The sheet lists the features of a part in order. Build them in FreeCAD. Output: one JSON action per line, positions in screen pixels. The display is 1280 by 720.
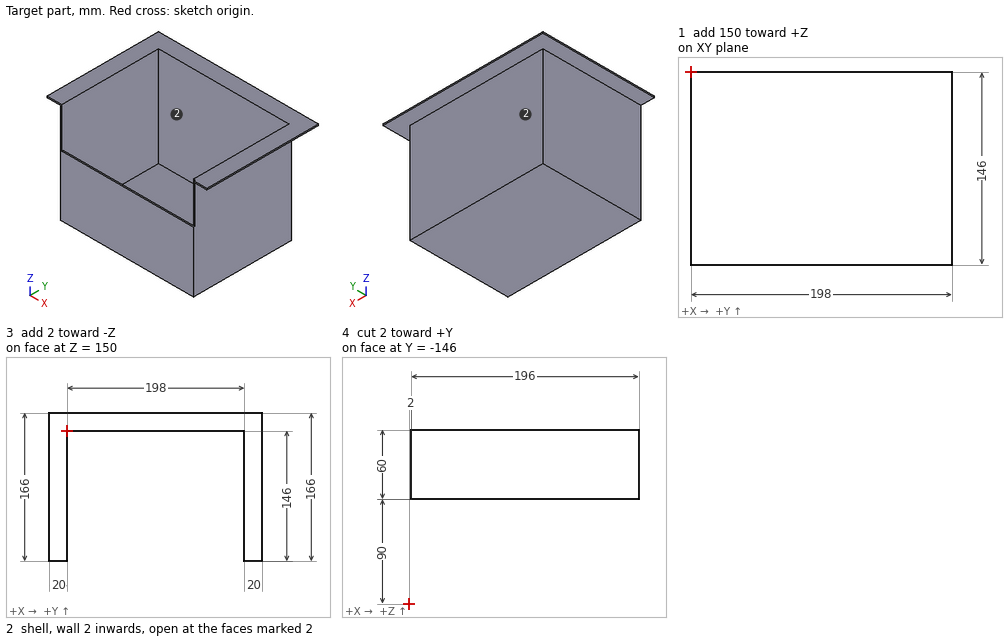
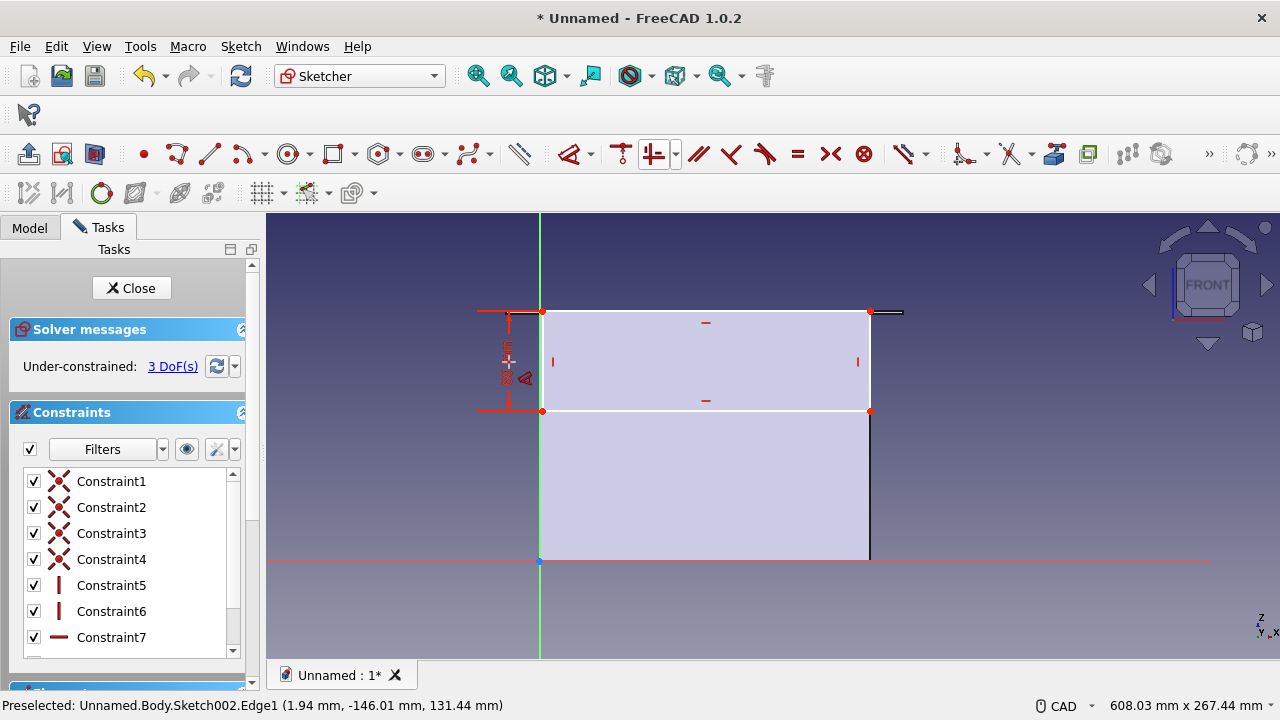
{"action": "scroll", "coordinate": [543, 311], "scroll_direction": "up", "scroll_amount": 13}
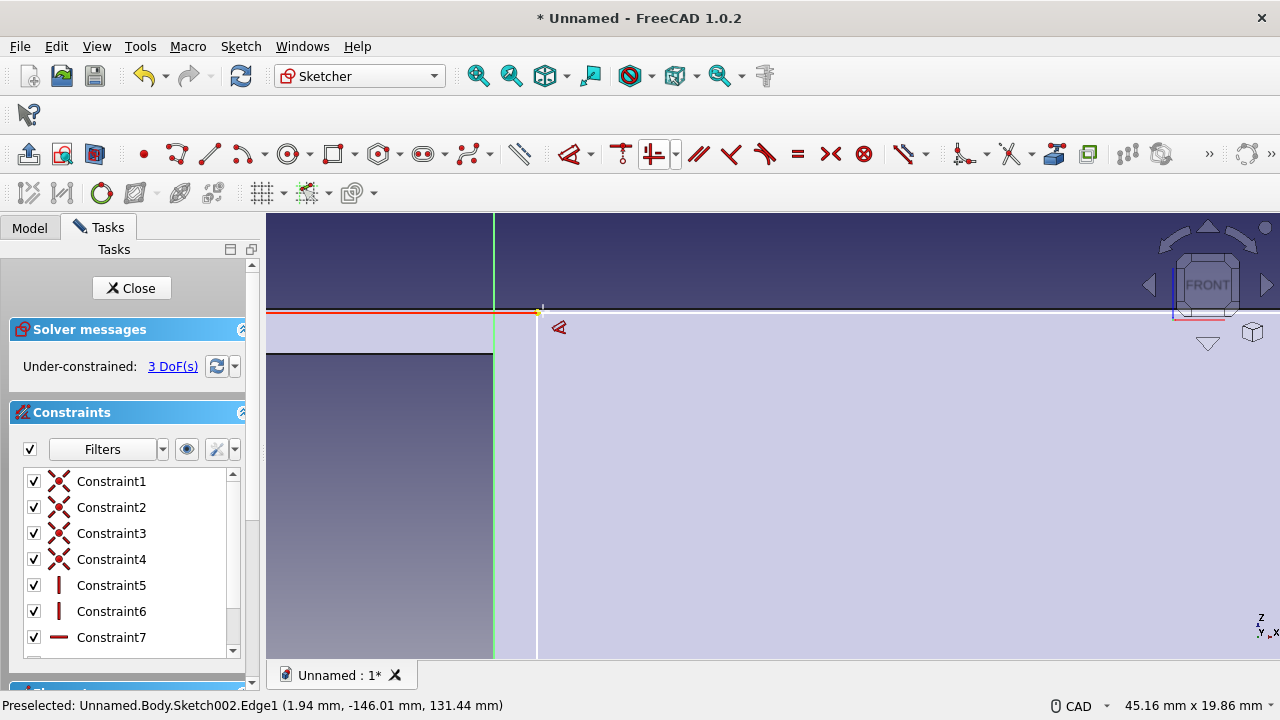
{"action": "left_click", "coordinate": [537, 313]}
{"action": "left_click", "coordinate": [515, 279]}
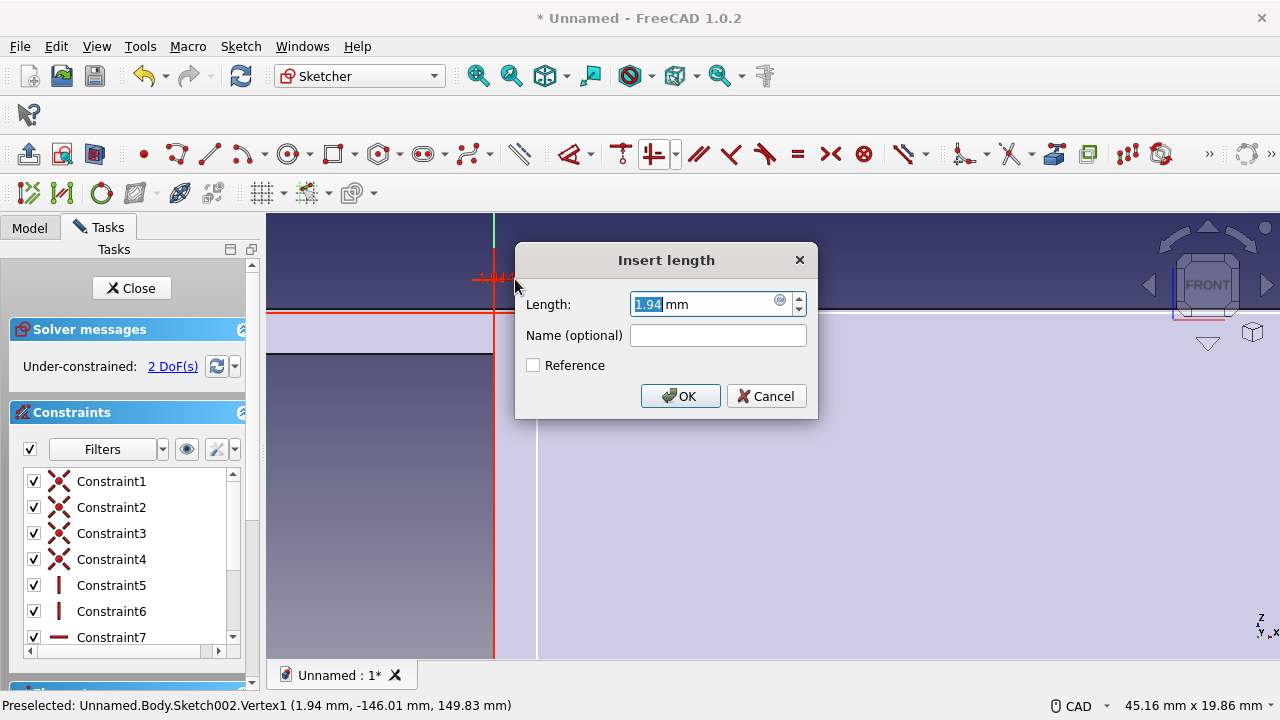
{"action": "type", "text": "2"}
{"action": "key", "text": "Return"}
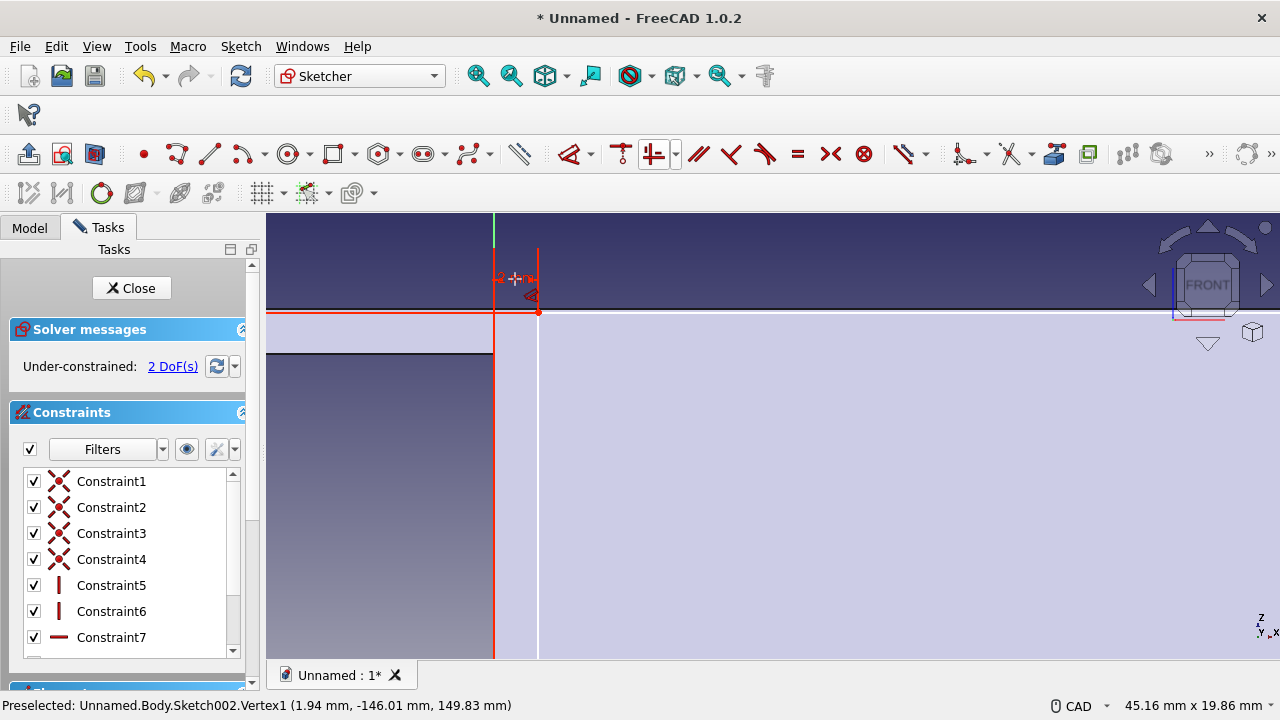
{"action": "scroll", "coordinate": [543, 311], "scroll_direction": "down", "scroll_amount": 13}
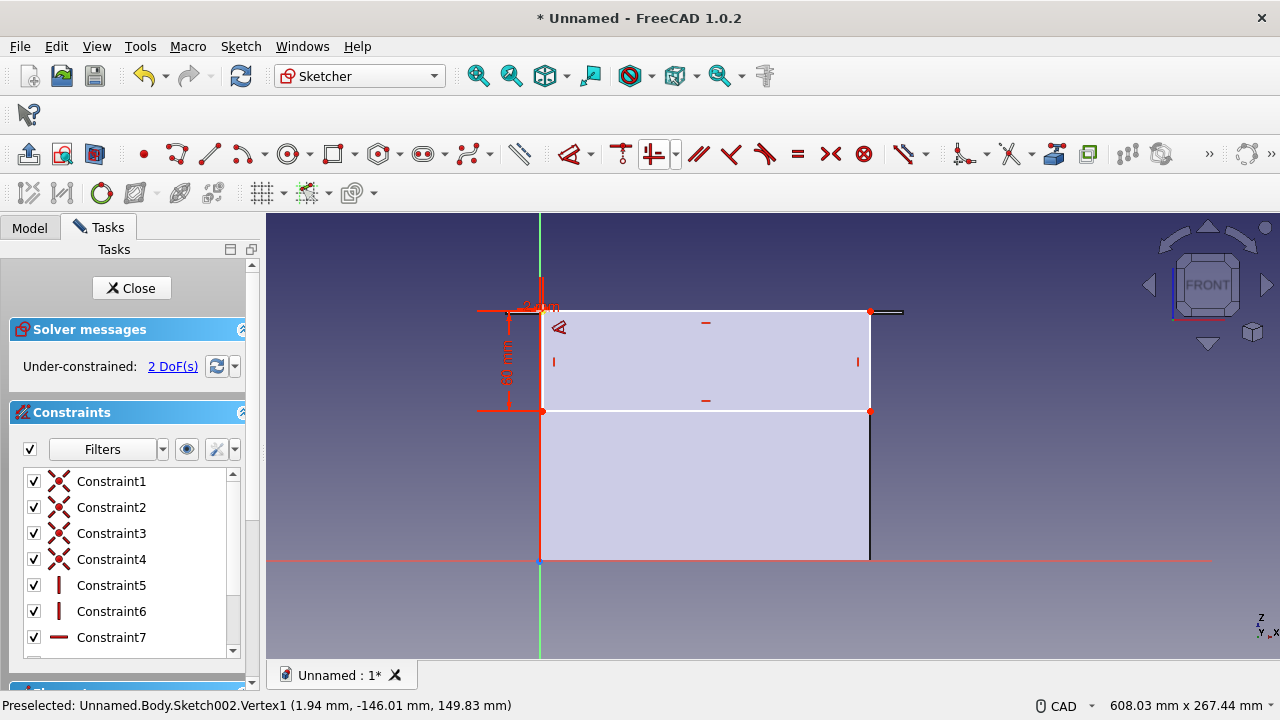
{"action": "left_click", "coordinate": [641, 411]}
{"action": "left_click", "coordinate": [706, 377]}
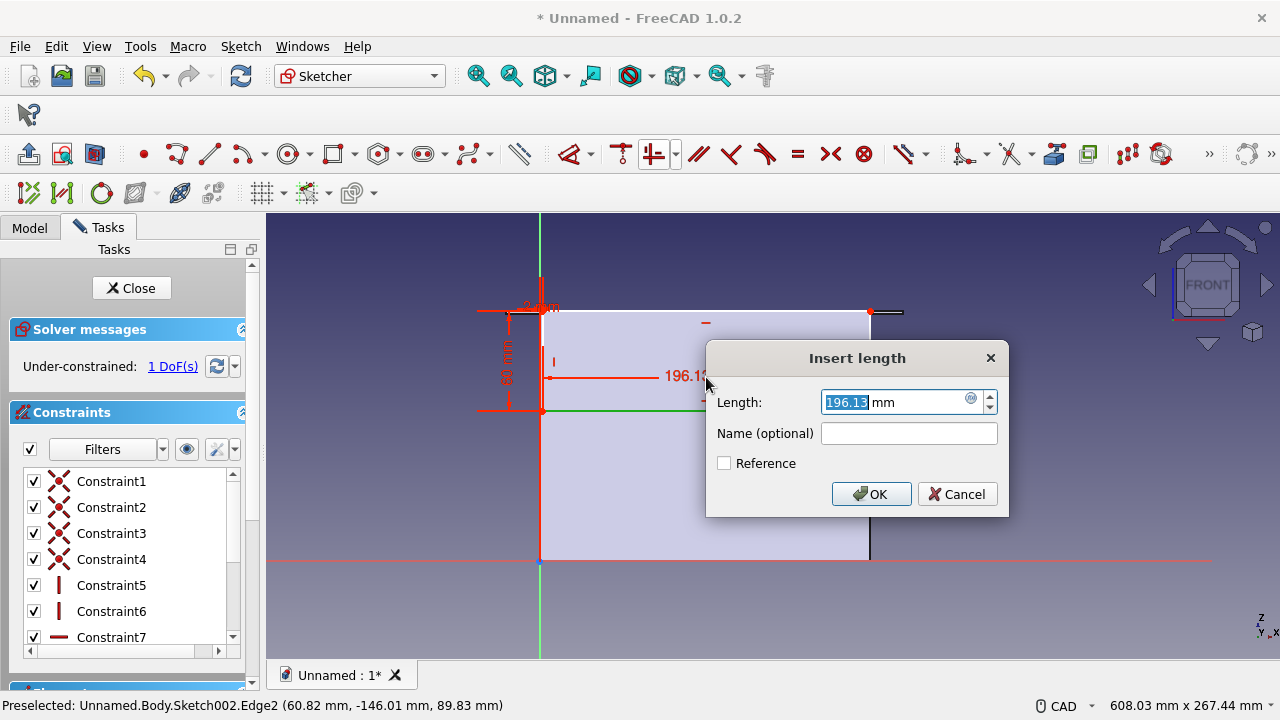
{"action": "type", "text": "196"}
{"action": "key", "text": "Return"}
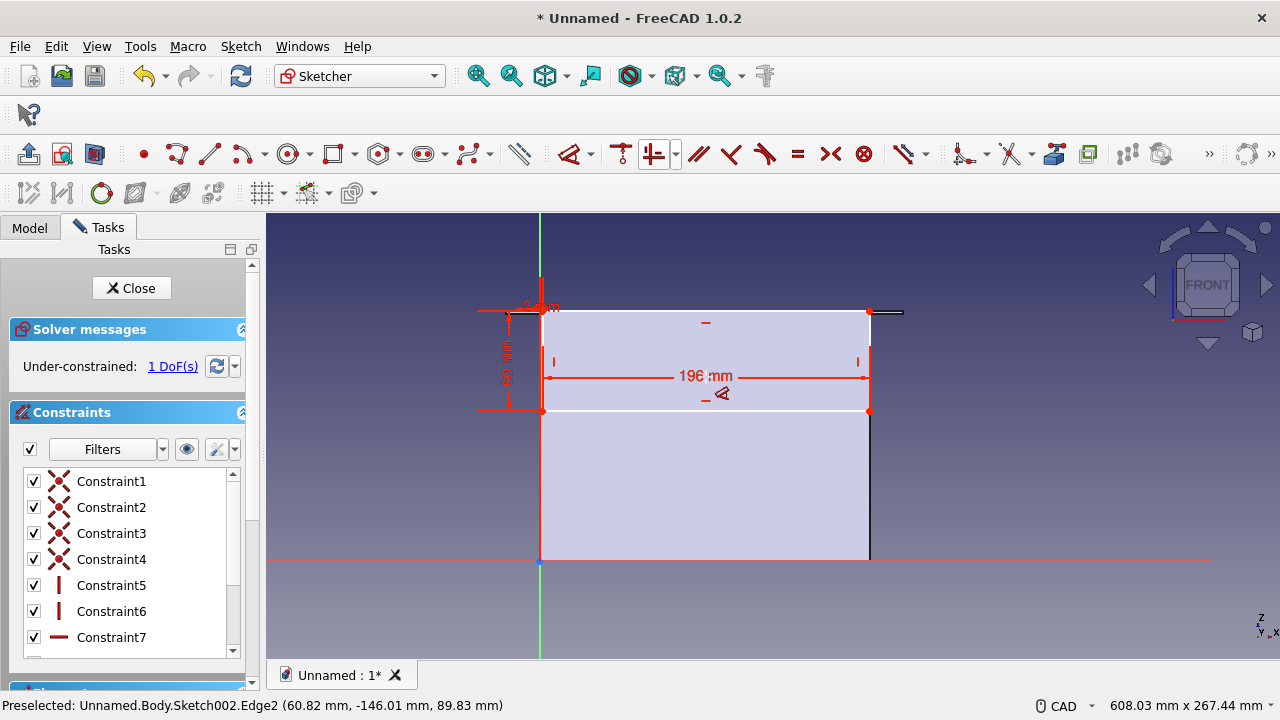
{"action": "left_click", "coordinate": [543, 411]}
{"action": "left_click", "coordinate": [506, 486]}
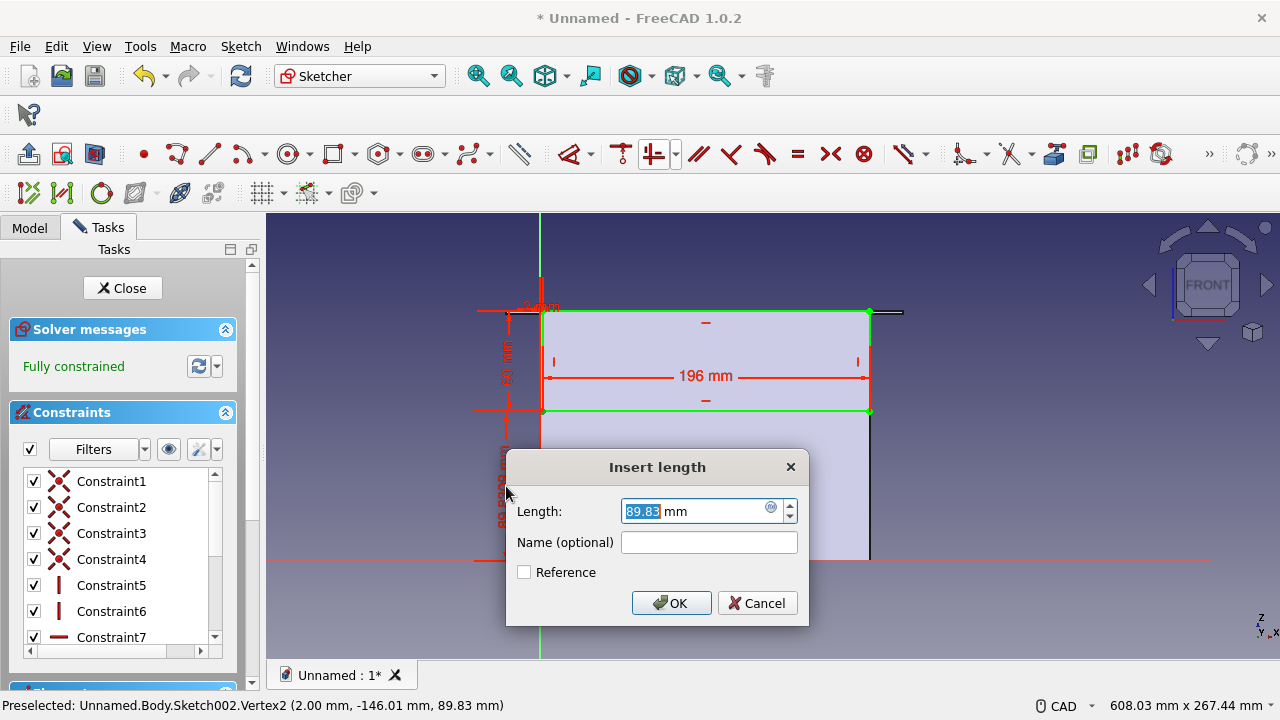
{"action": "type", "text": "90"}
{"action": "key", "text": "Return"}
{"action": "key", "text": "Escape"}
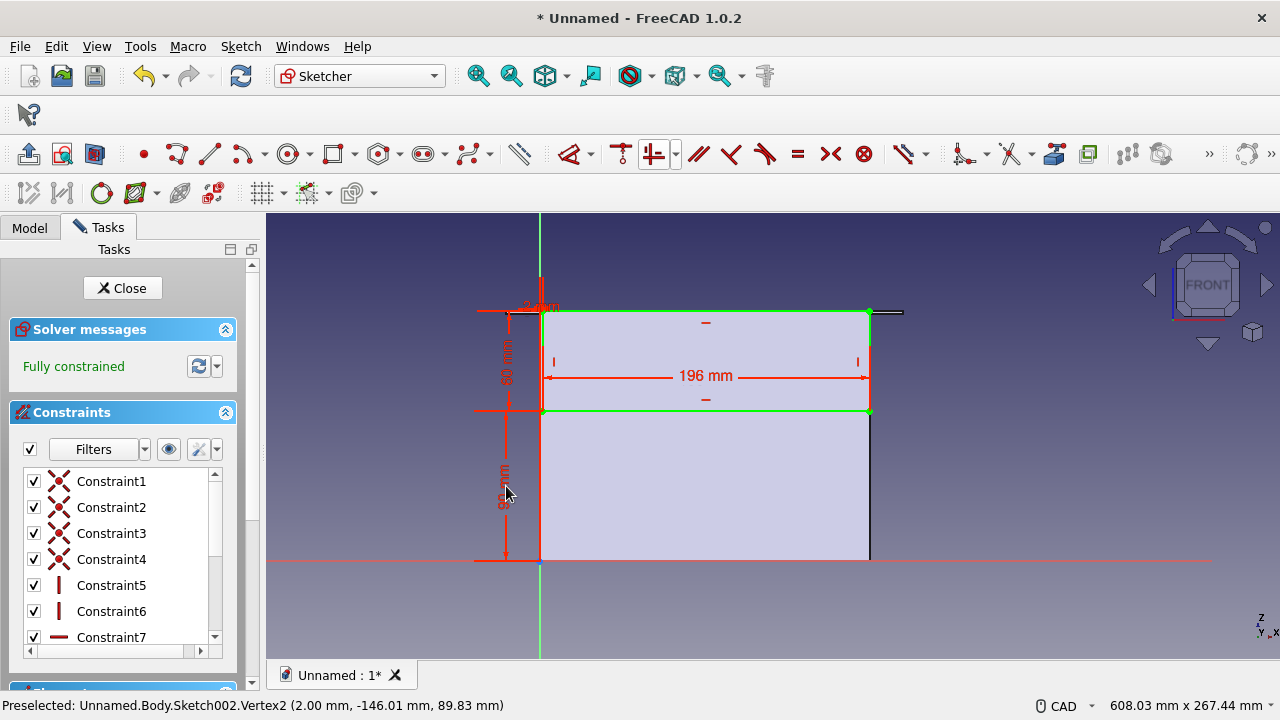
{"action": "left_click", "coordinate": [123, 288]}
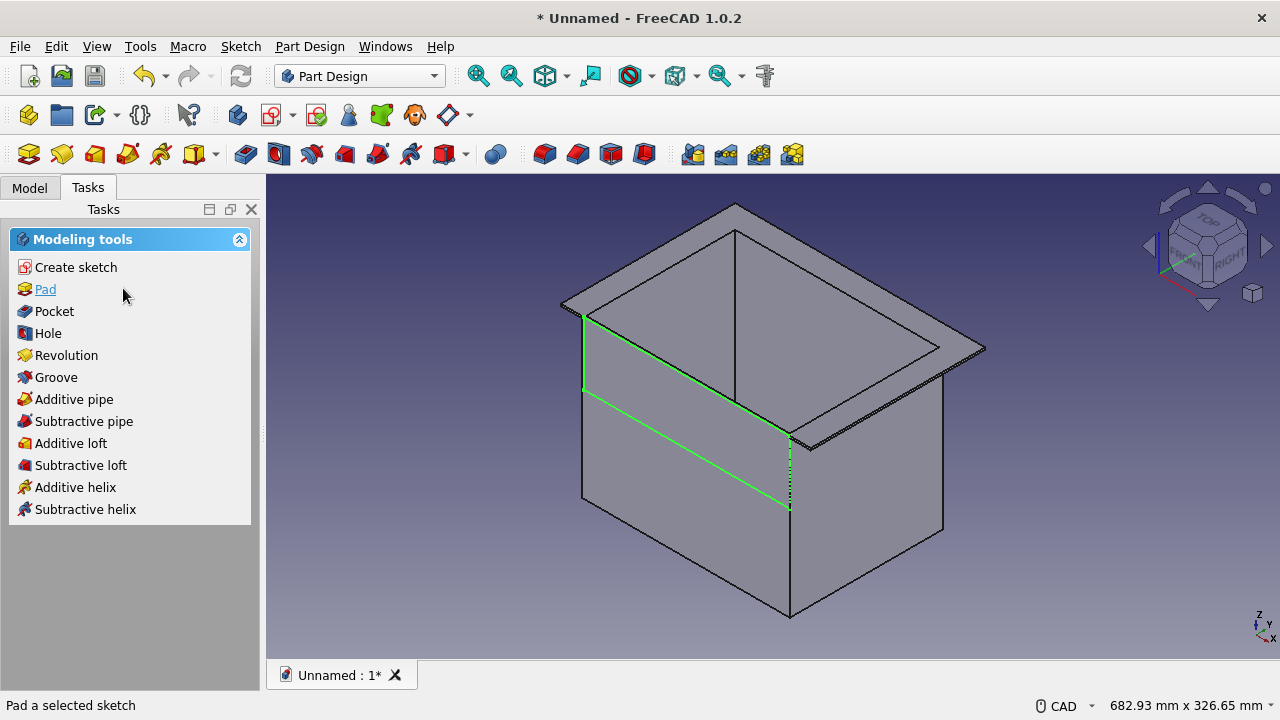
{"action": "left_click", "coordinate": [246, 154]}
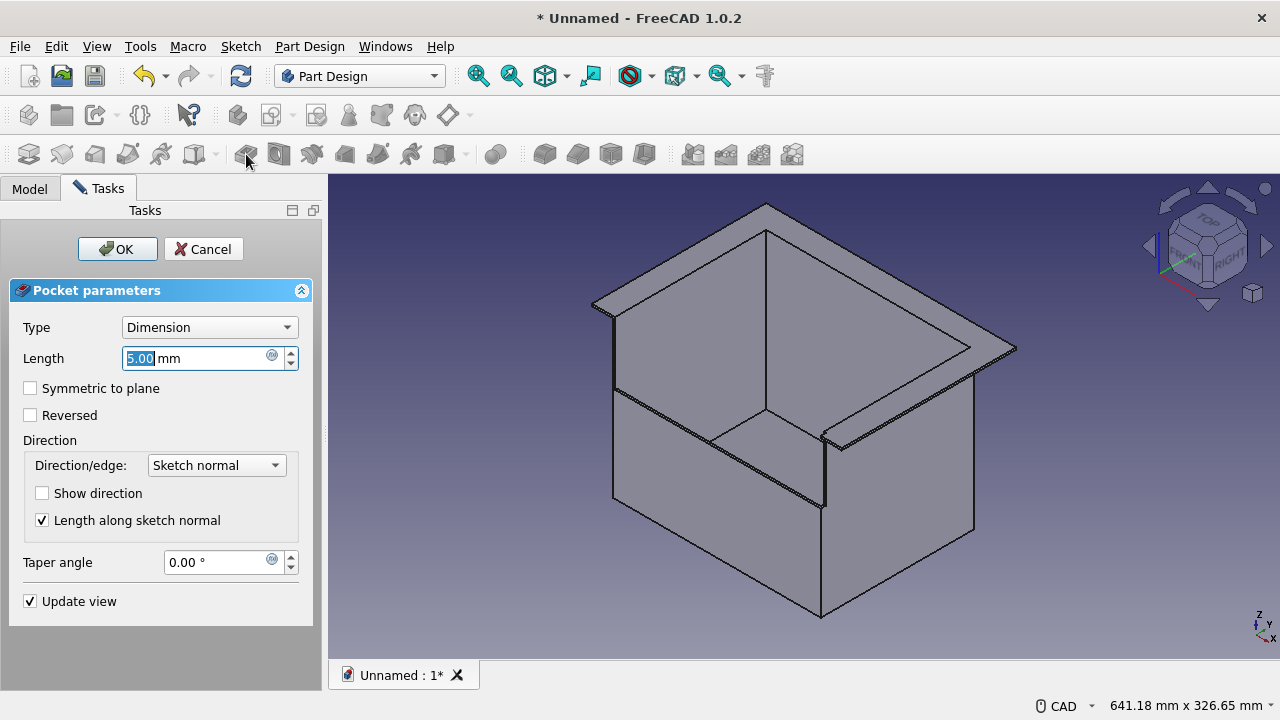
{"action": "type", "text": "2"}
{"action": "key", "text": "Tab"}